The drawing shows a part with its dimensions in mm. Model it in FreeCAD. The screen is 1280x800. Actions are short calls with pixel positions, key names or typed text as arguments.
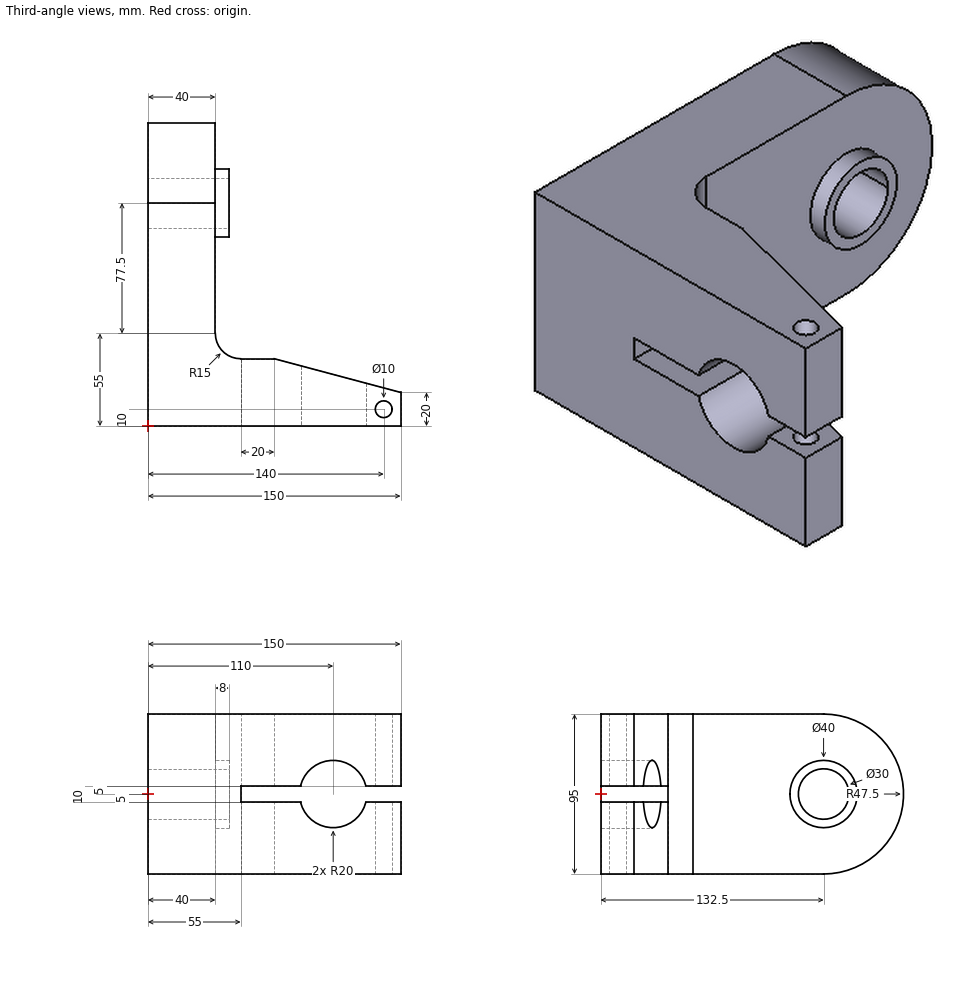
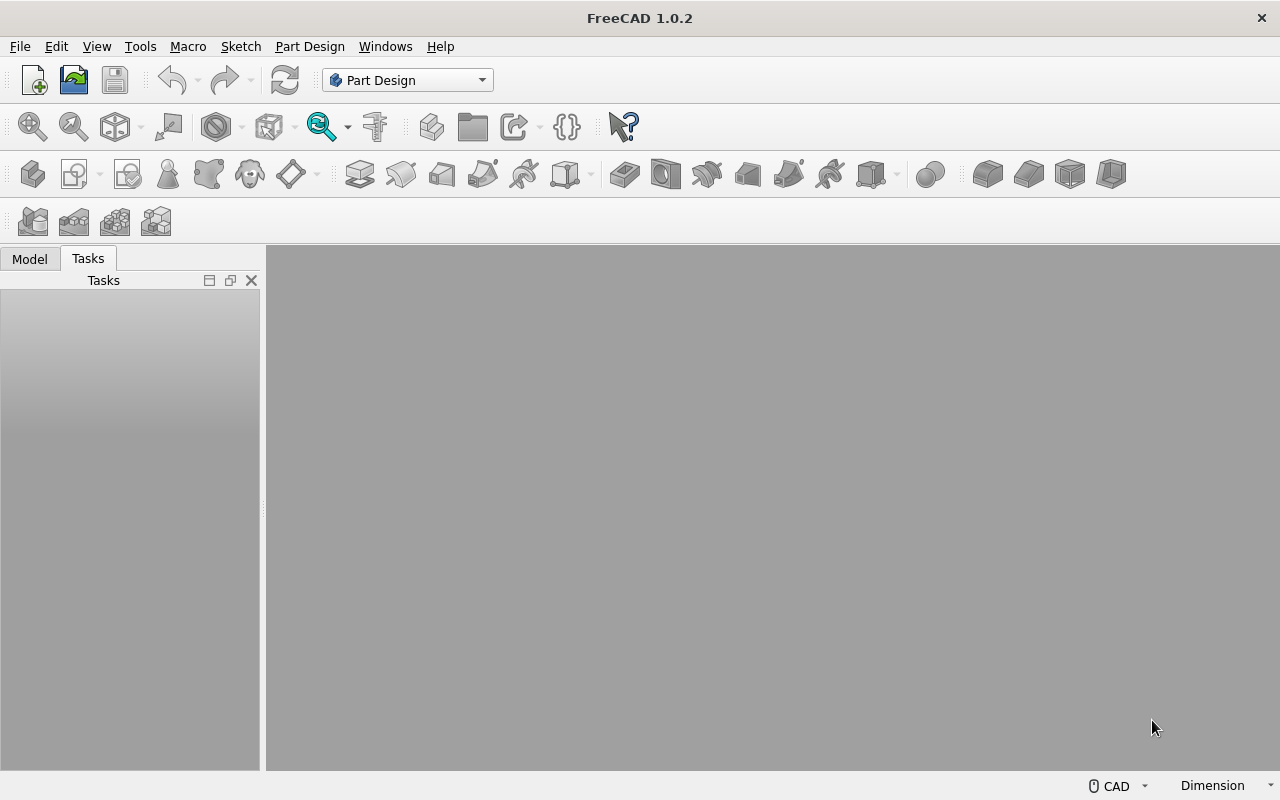
click(33, 80)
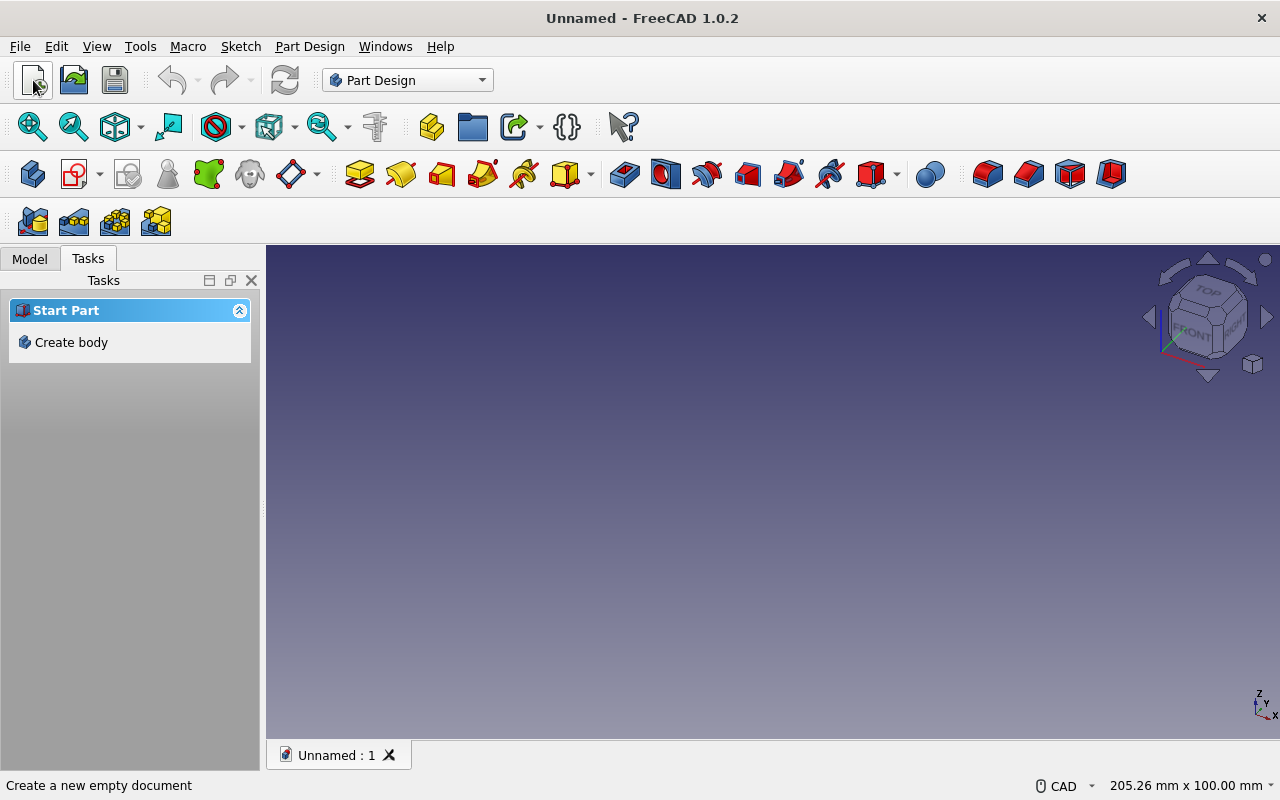
click(74, 174)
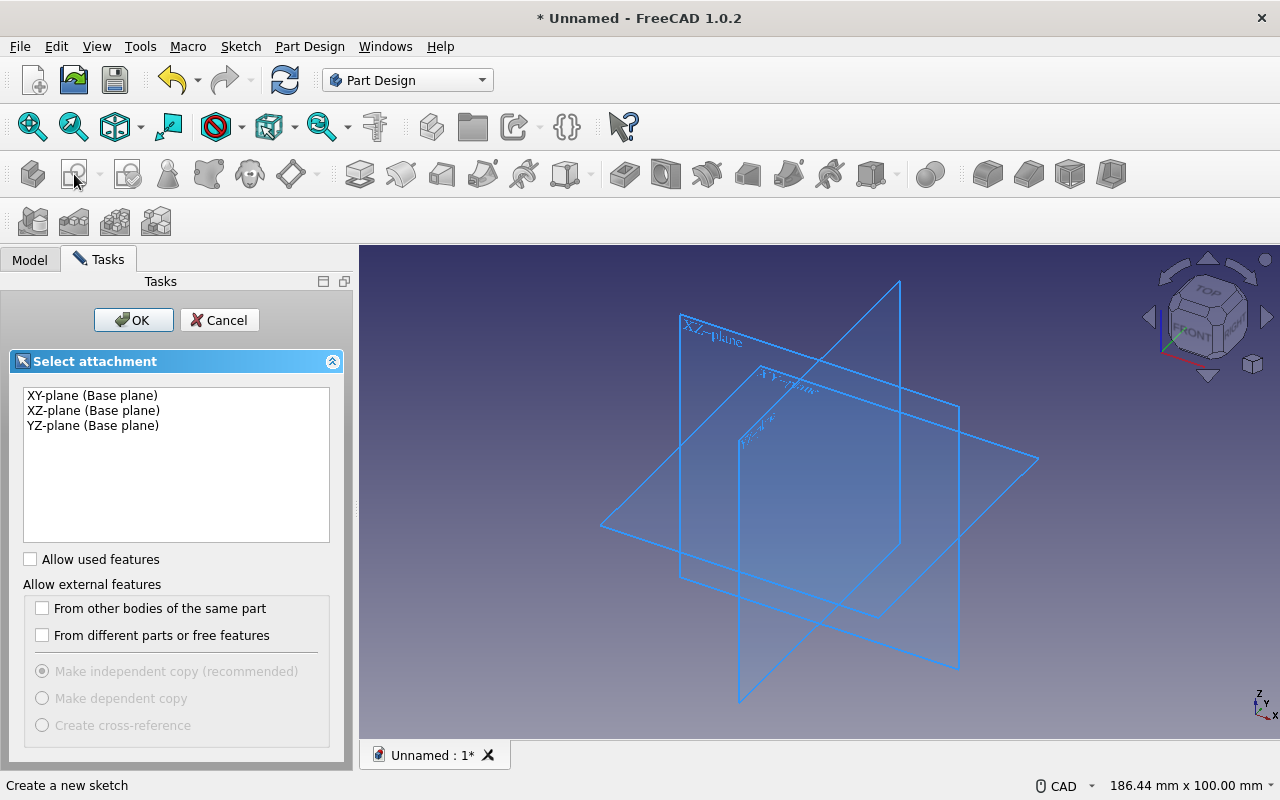
click(84, 396)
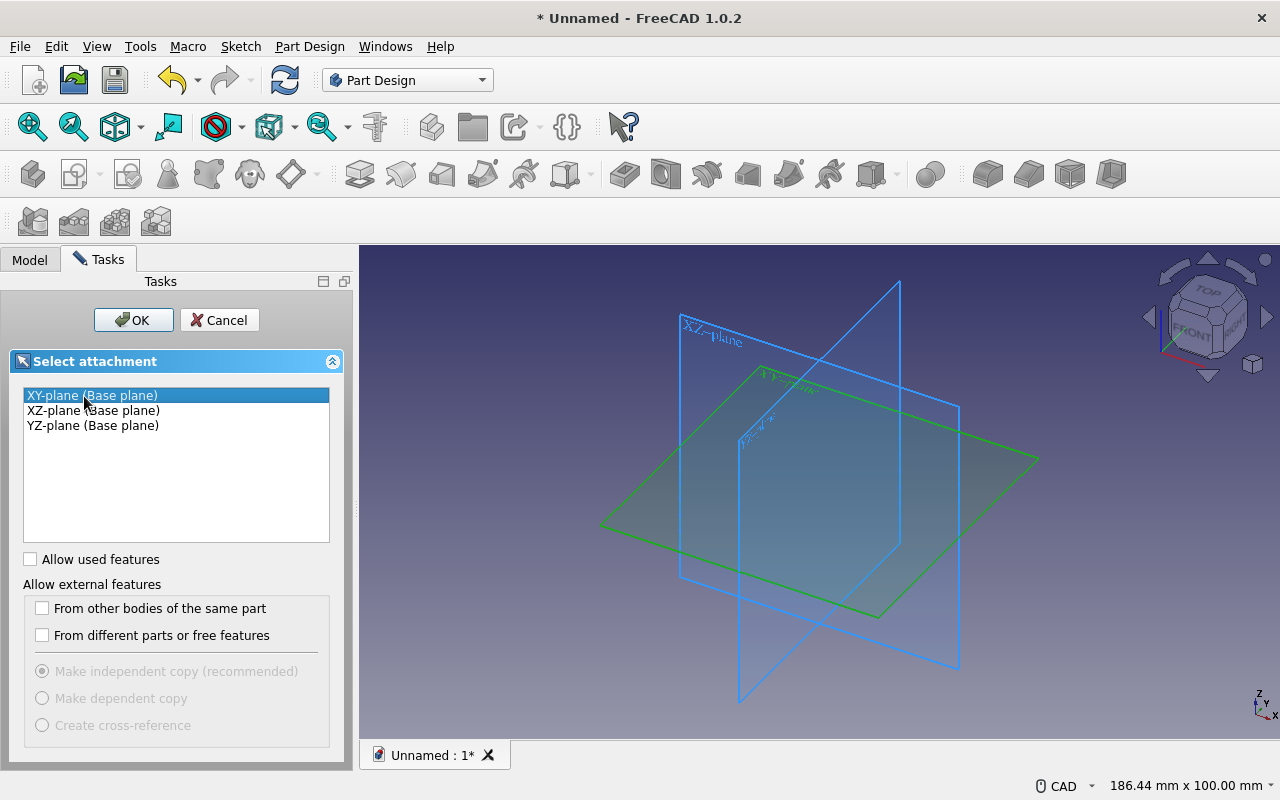
click(134, 320)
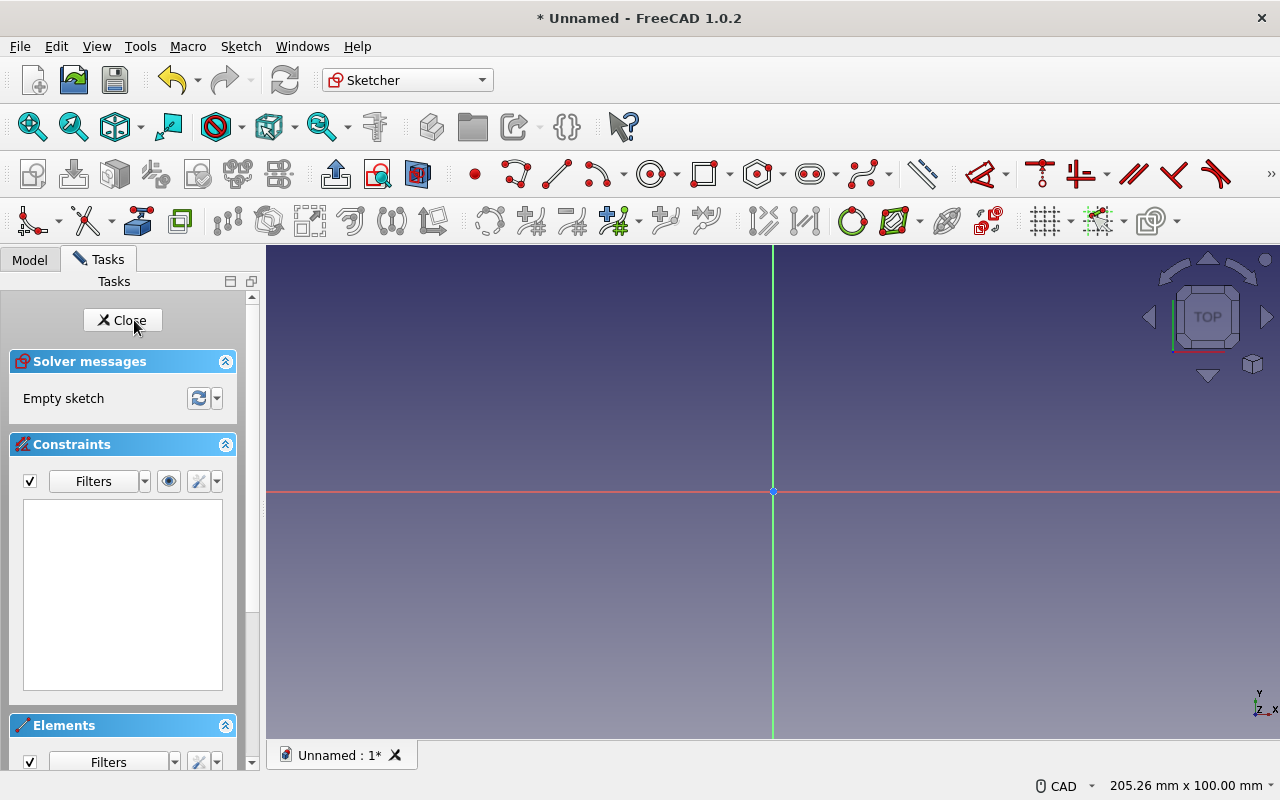
scroll(346, 711, down, 4)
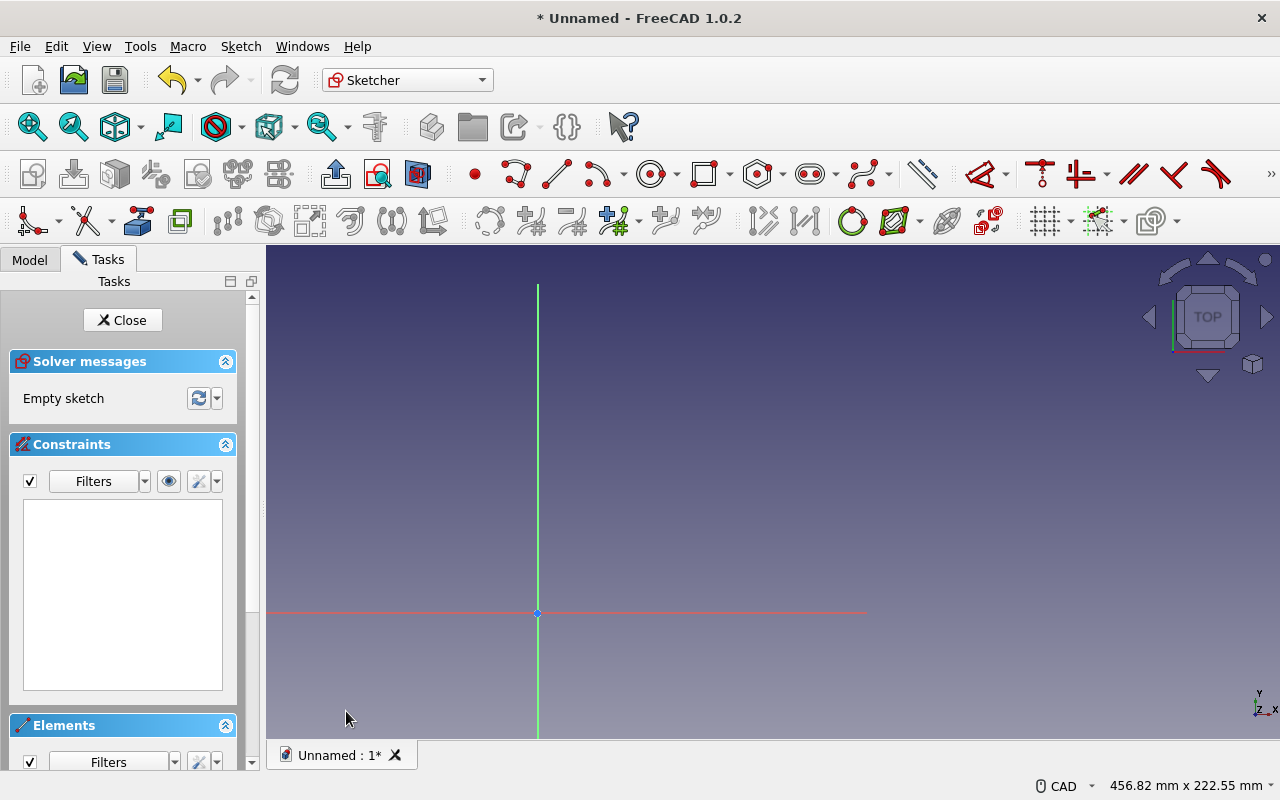
click(516, 174)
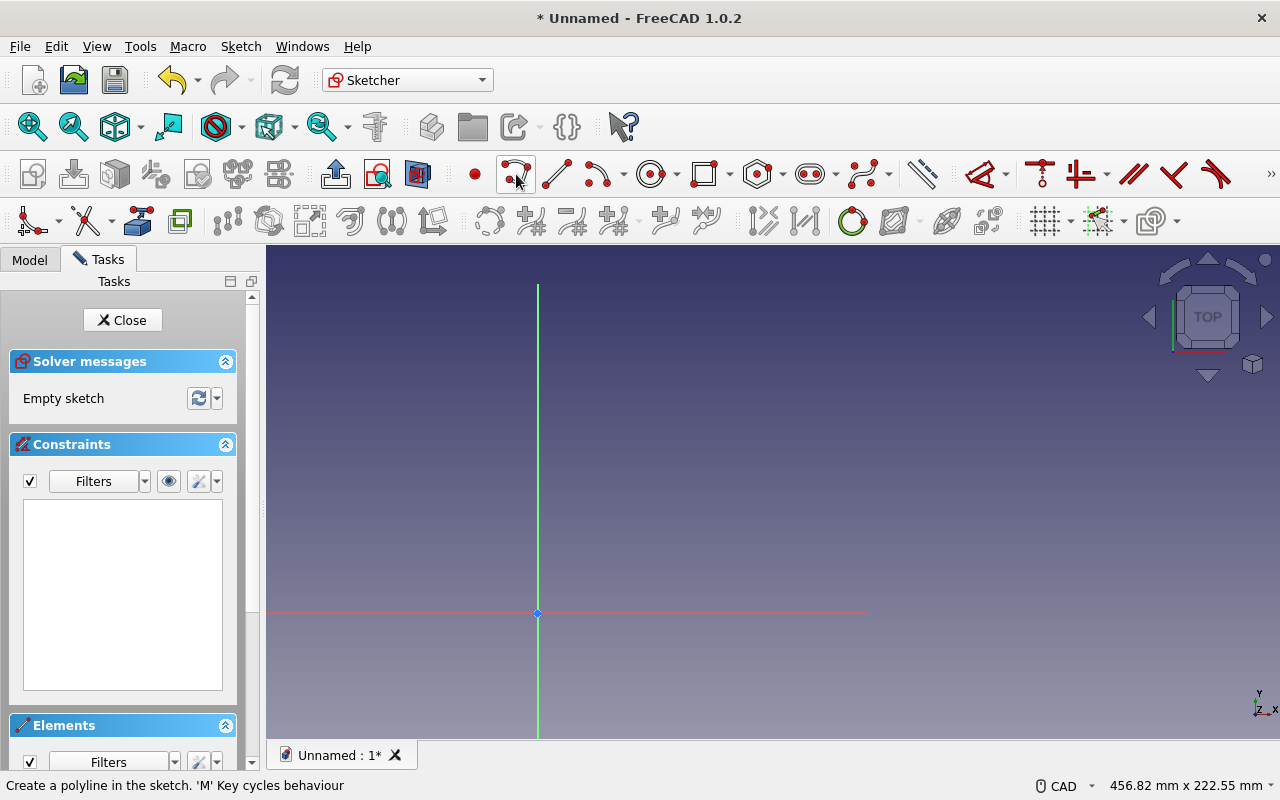
click(627, 491)
click(627, 319)
click(538, 319)
click(538, 613)
click(871, 604)
click(871, 569)
click(704, 524)
click(660, 524)
right_click(660, 524)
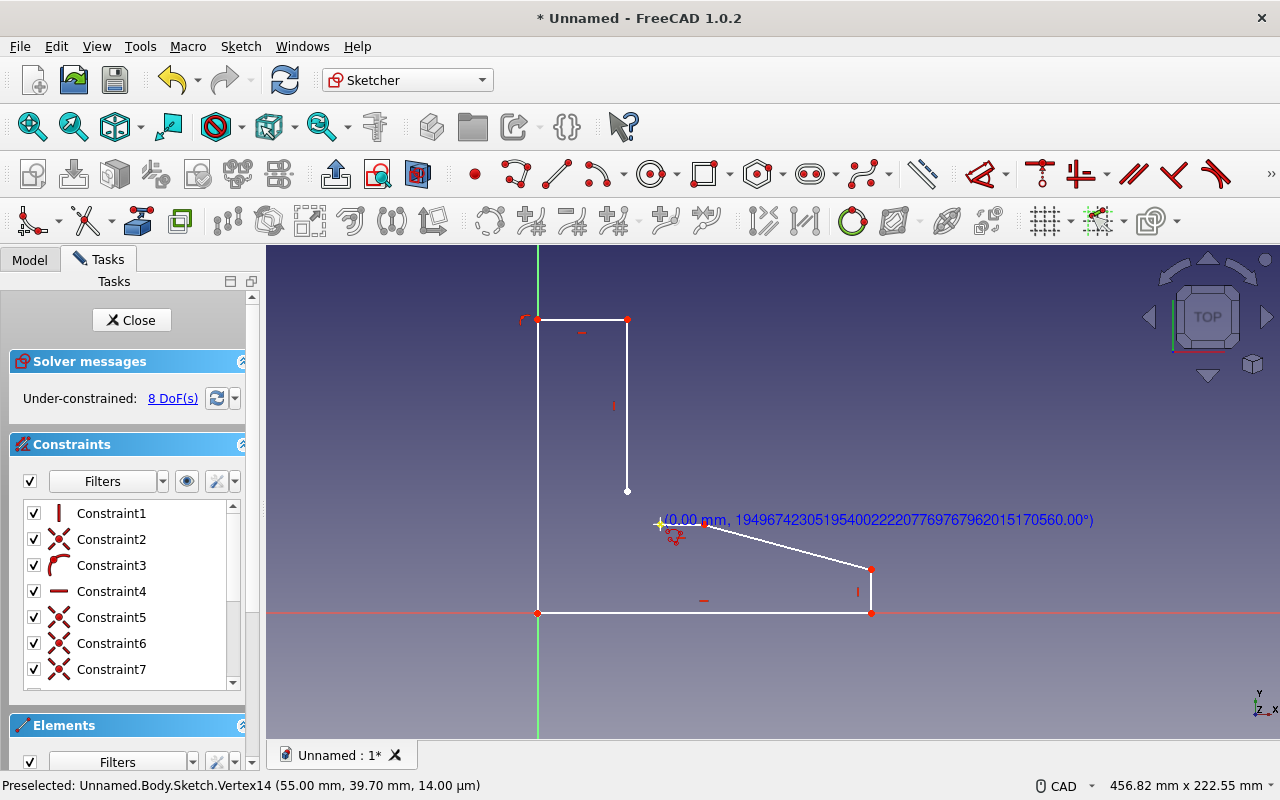
click(624, 174)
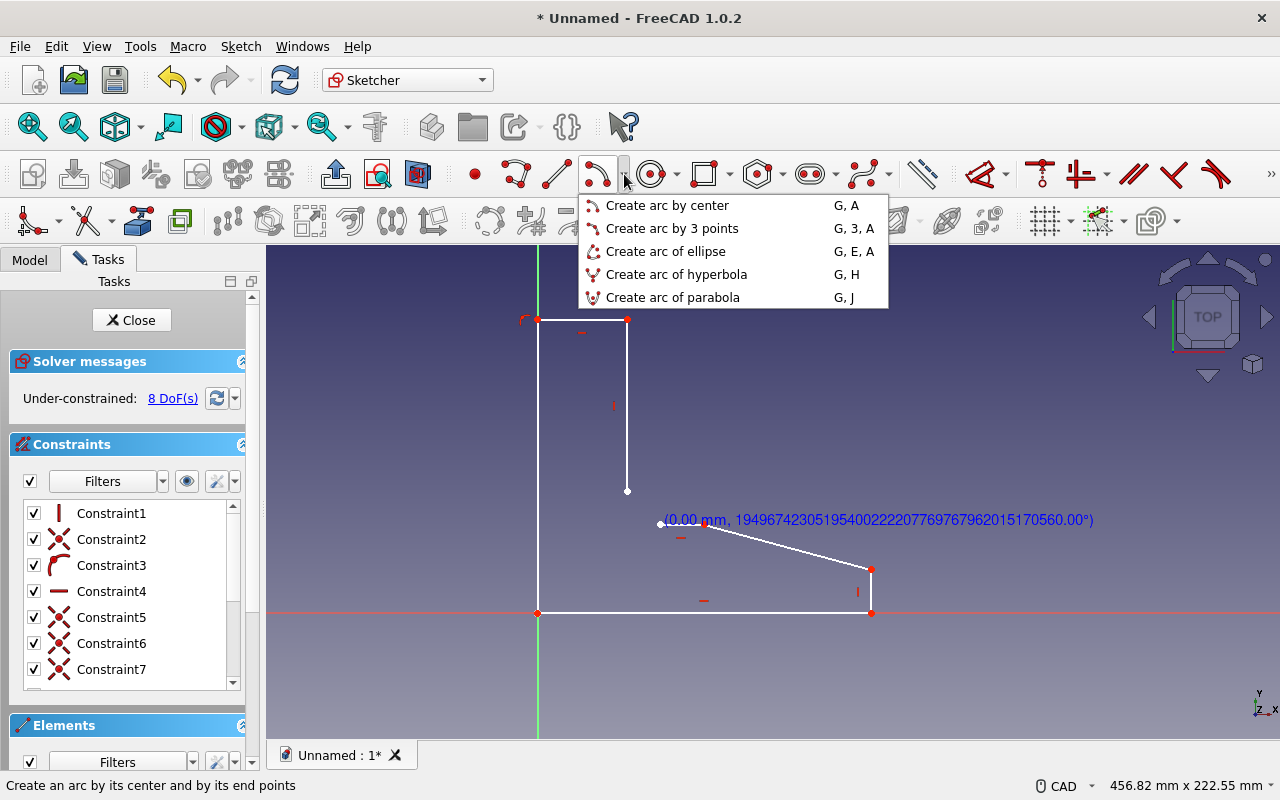
click(734, 228)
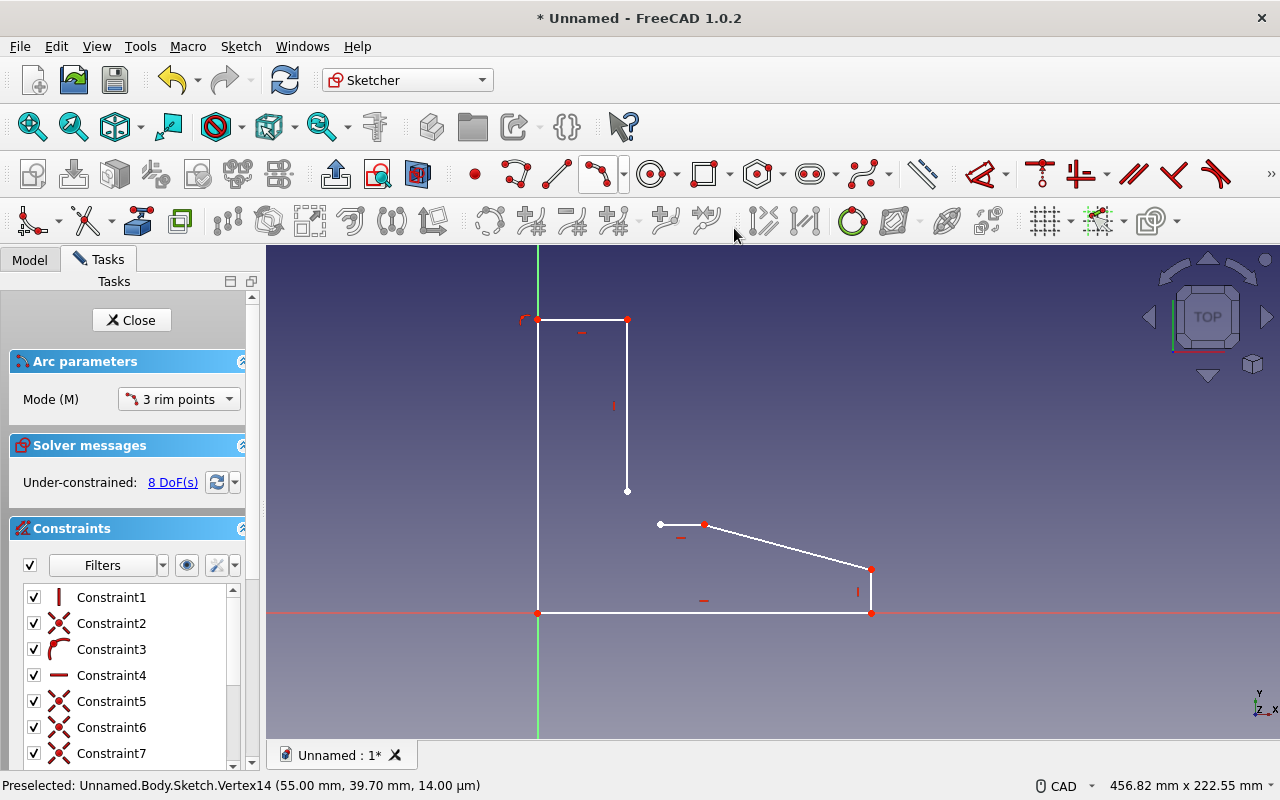
click(660, 525)
click(627, 492)